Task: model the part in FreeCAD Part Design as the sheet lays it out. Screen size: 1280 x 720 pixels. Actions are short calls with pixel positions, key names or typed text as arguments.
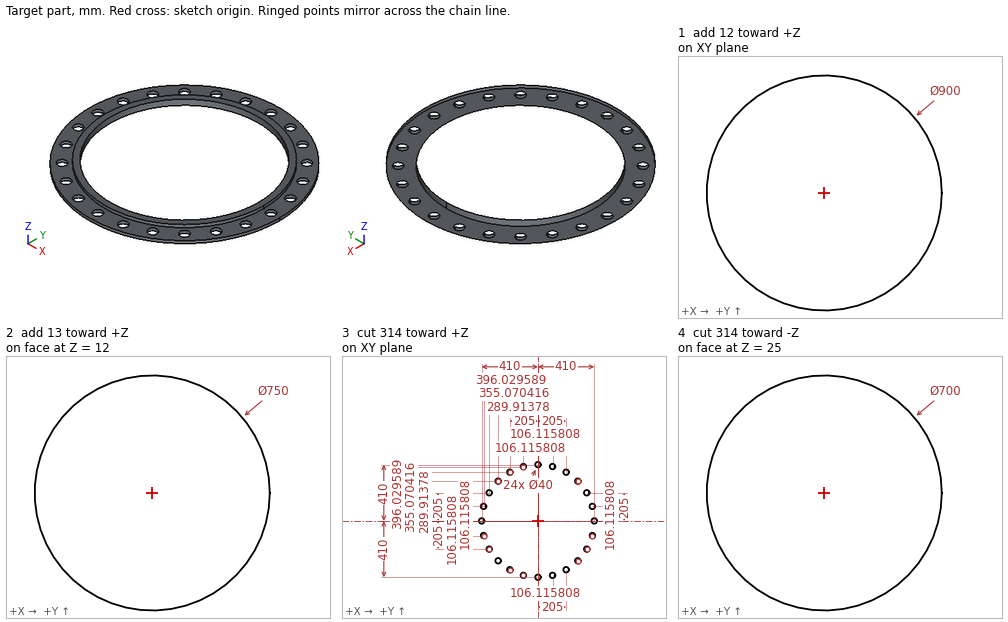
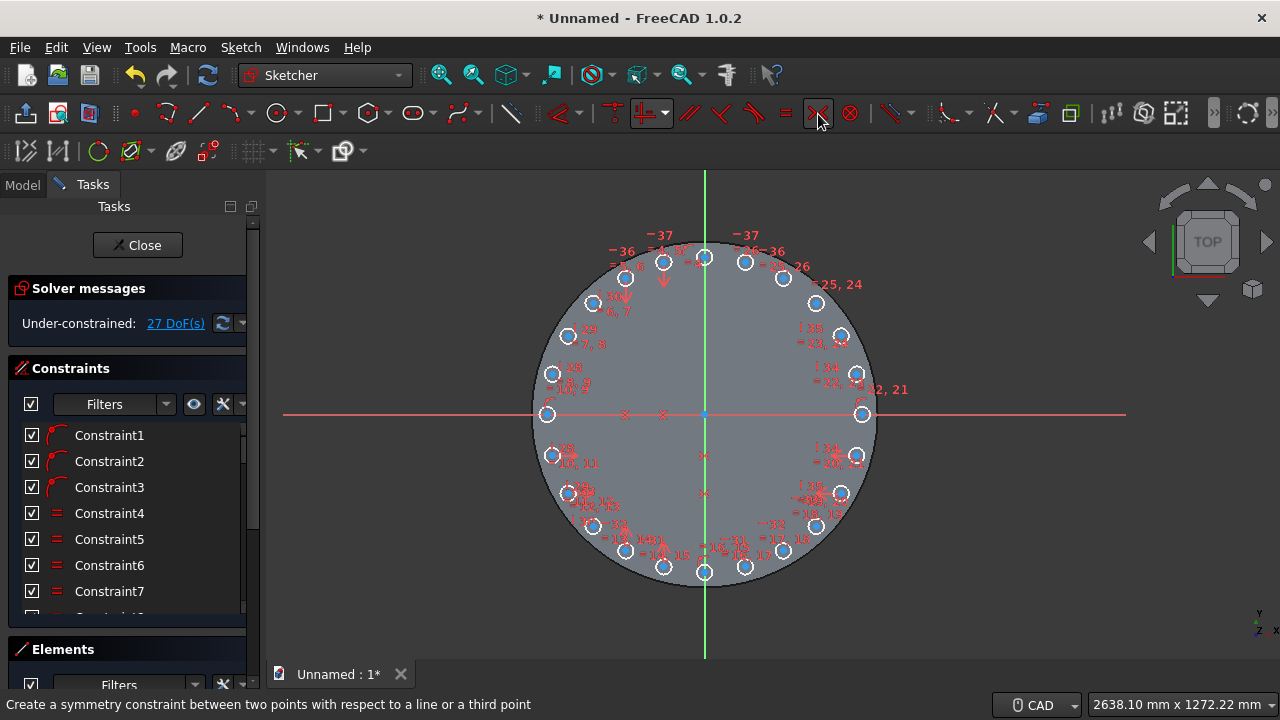
click(593, 303)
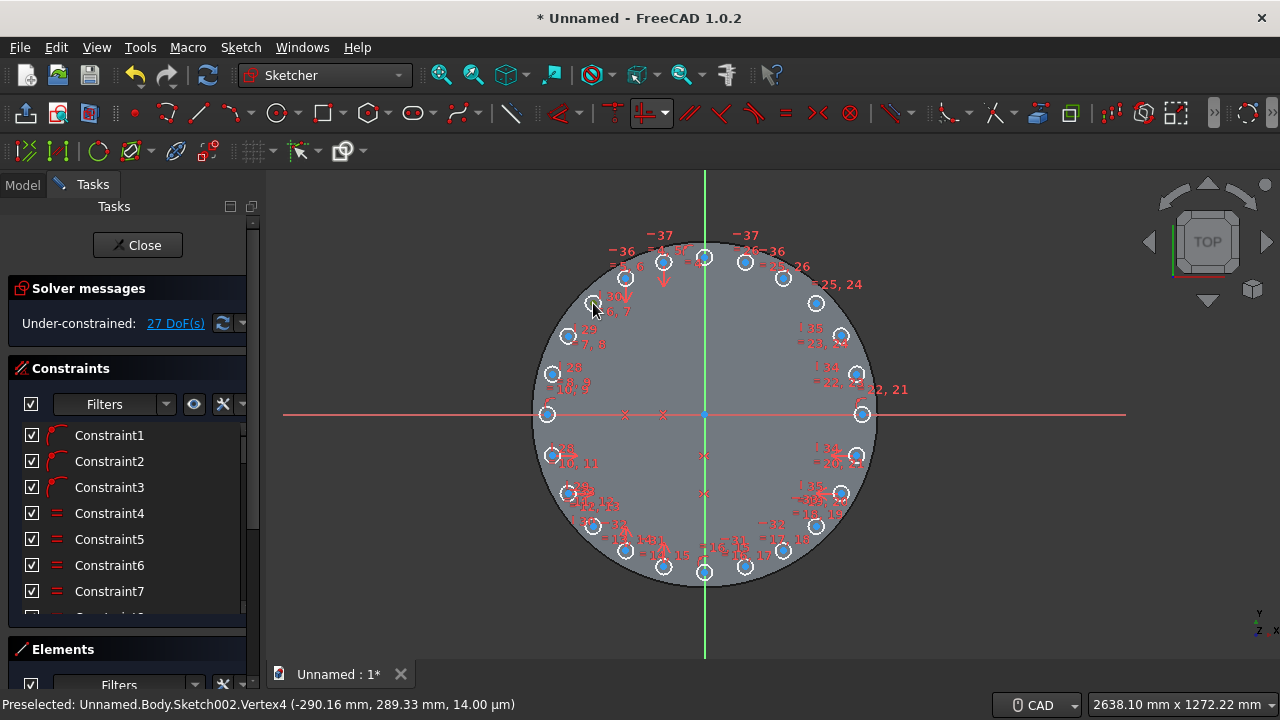
click(816, 303)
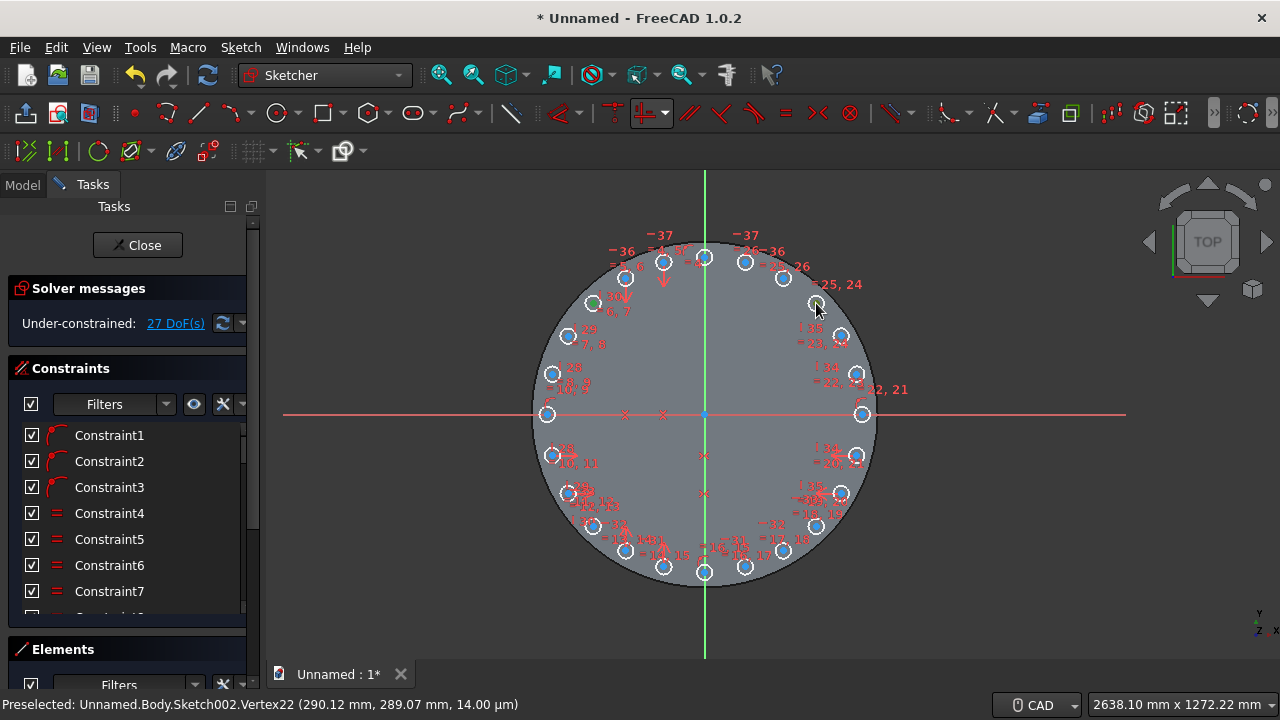
click(705, 507)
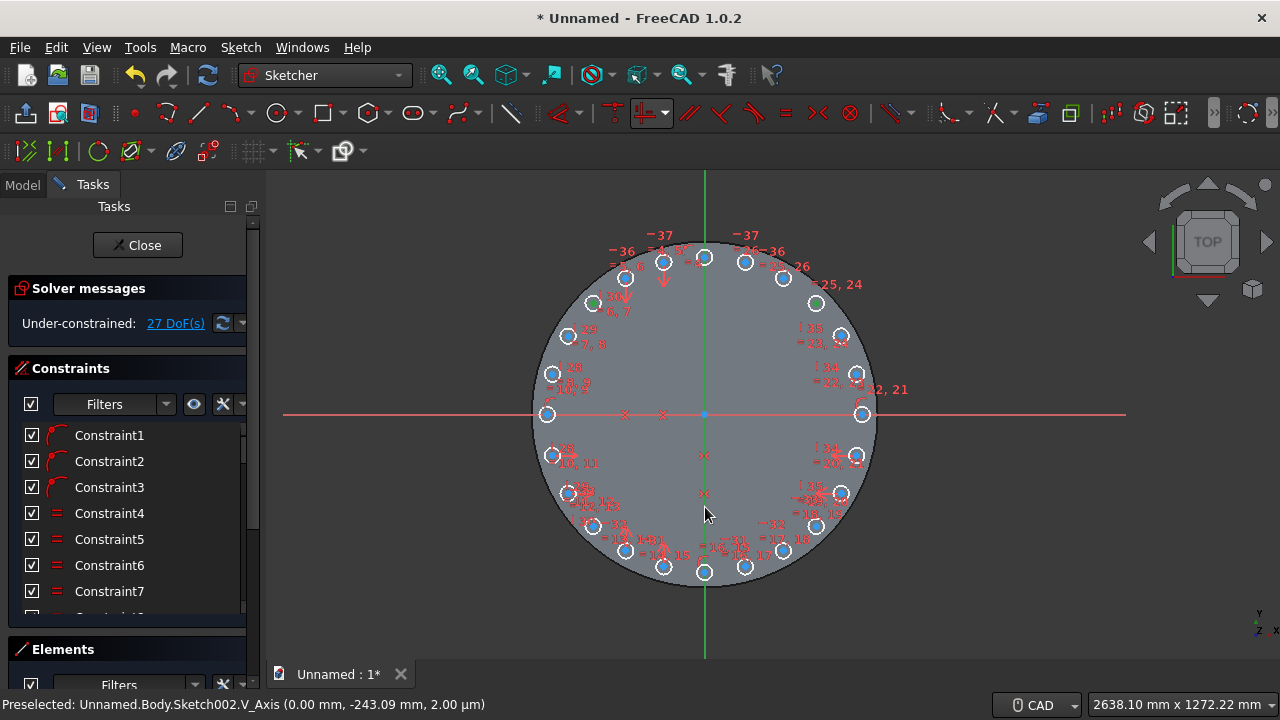
click(818, 114)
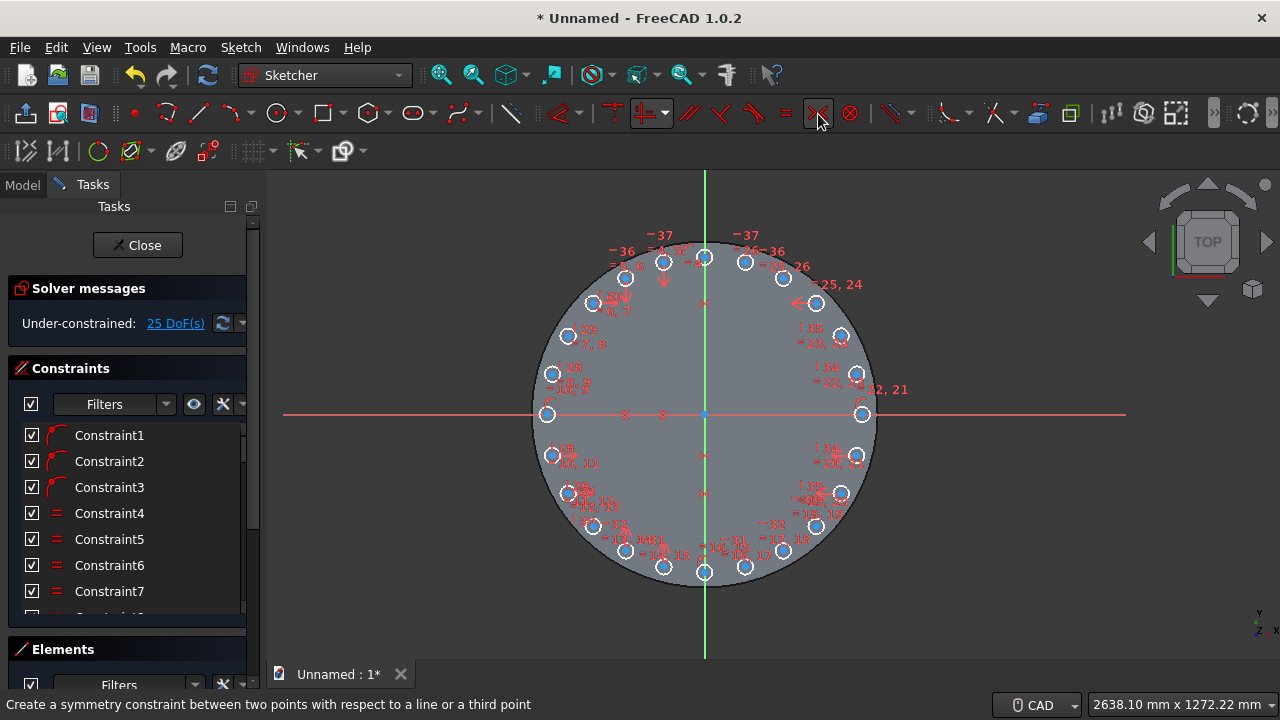
click(816, 526)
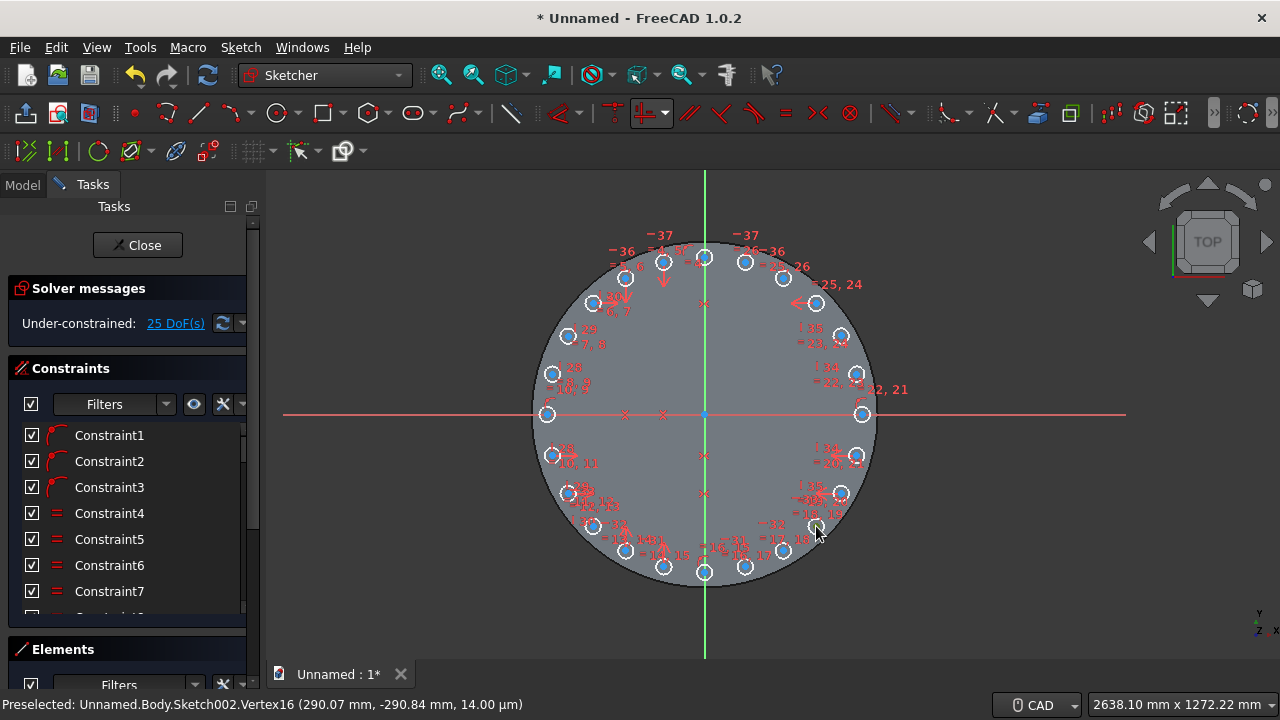
click(816, 303)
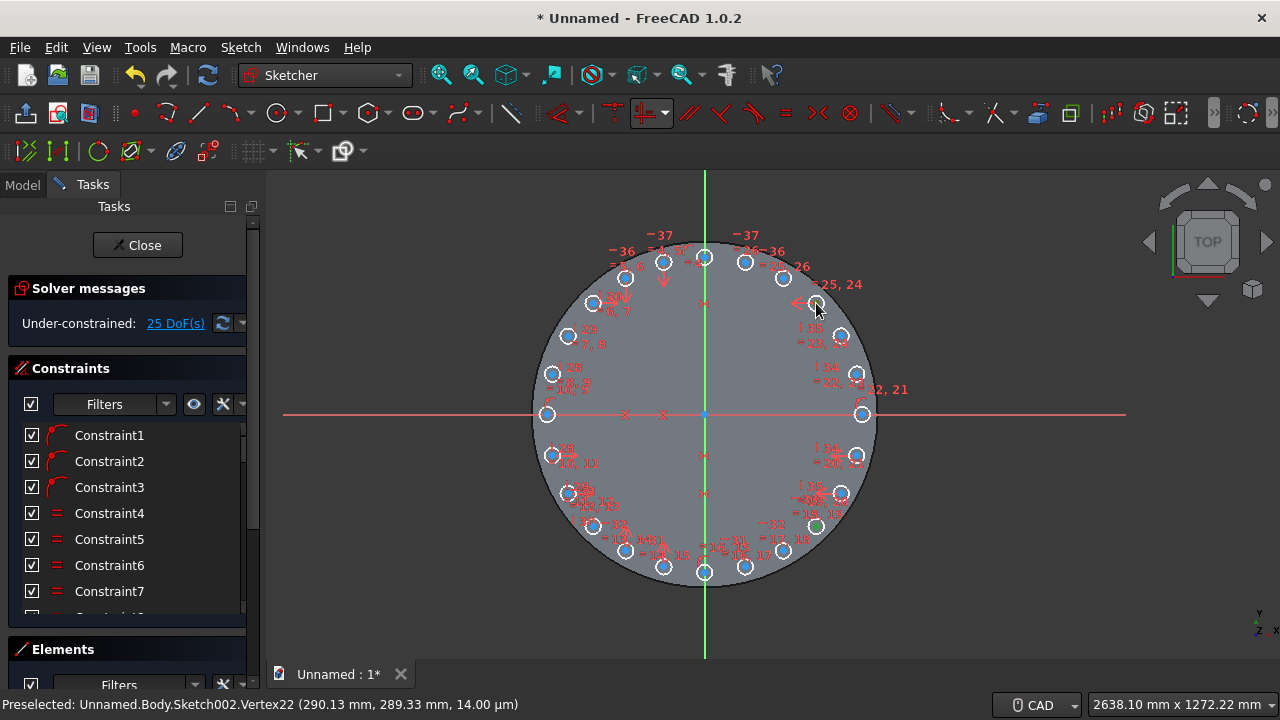
click(353, 415)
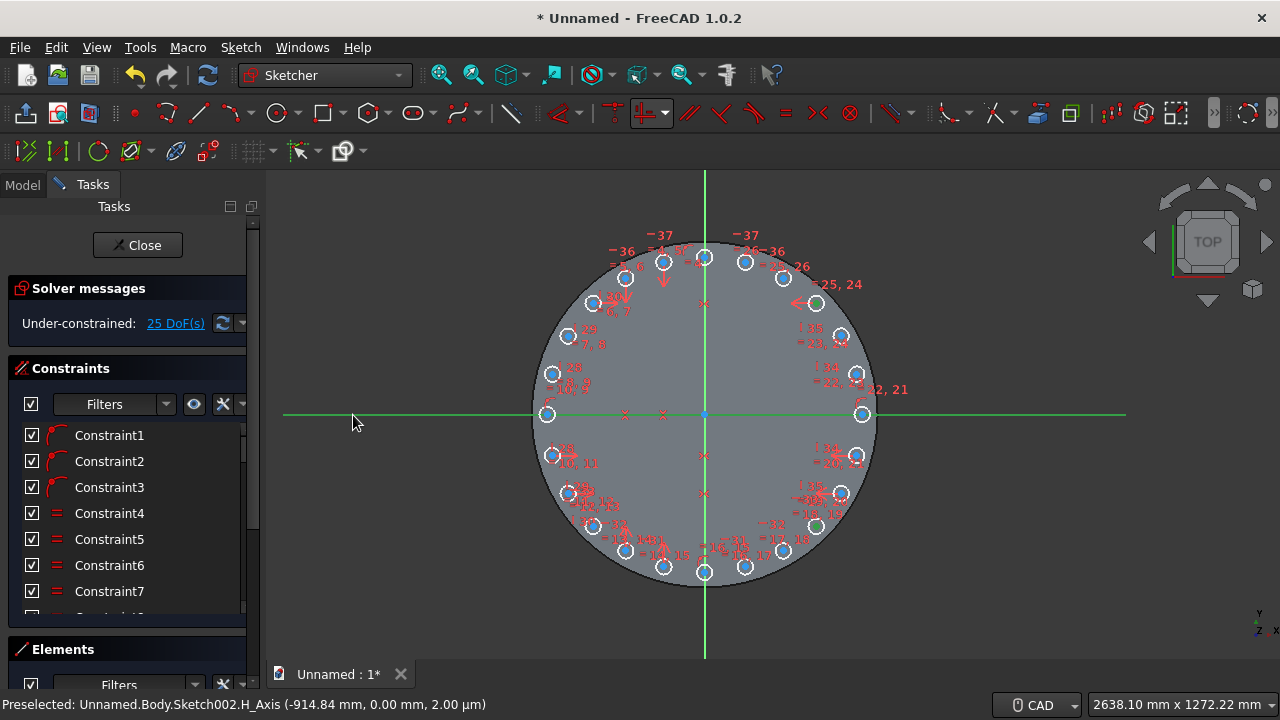
click(818, 114)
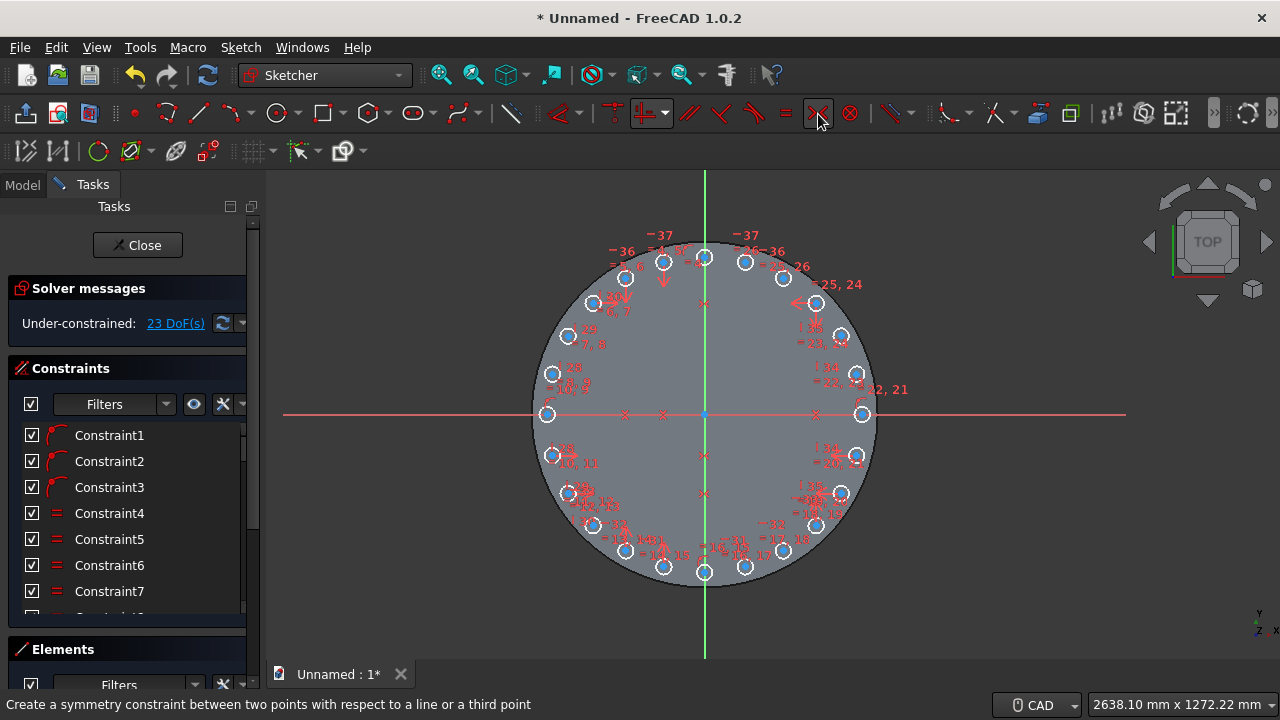
click(558, 114)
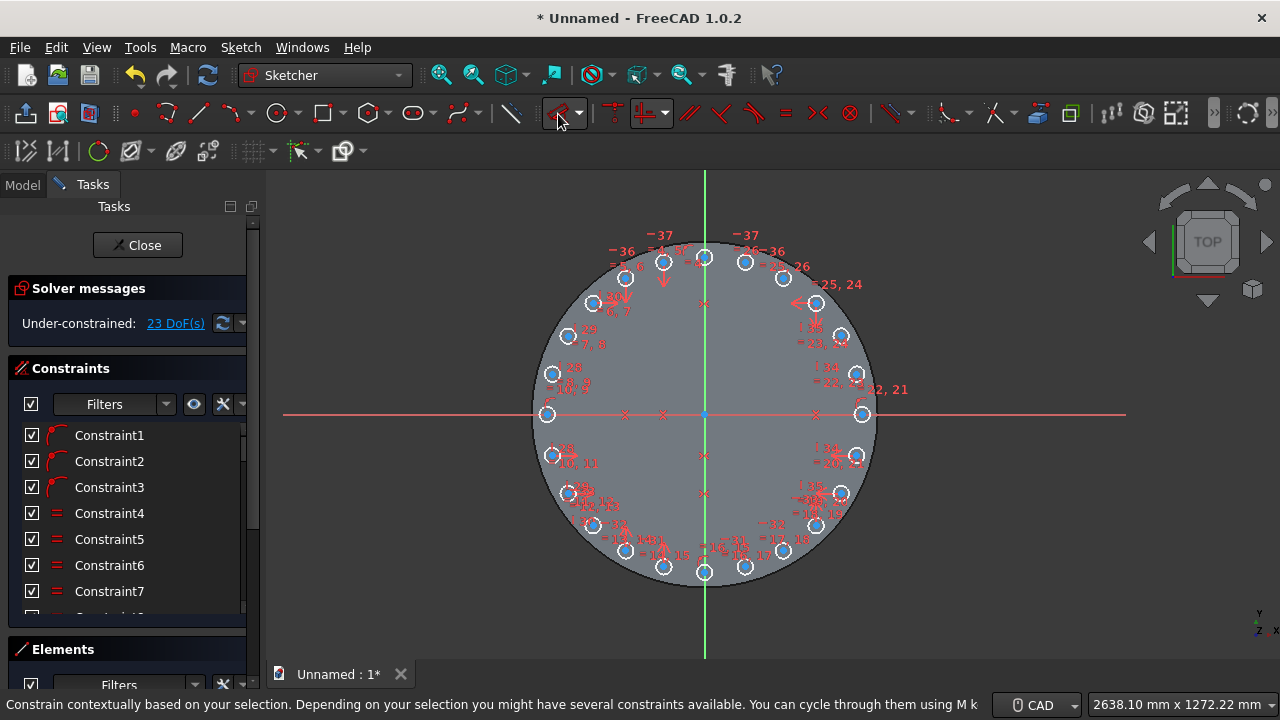
scroll(705, 250, up, 5)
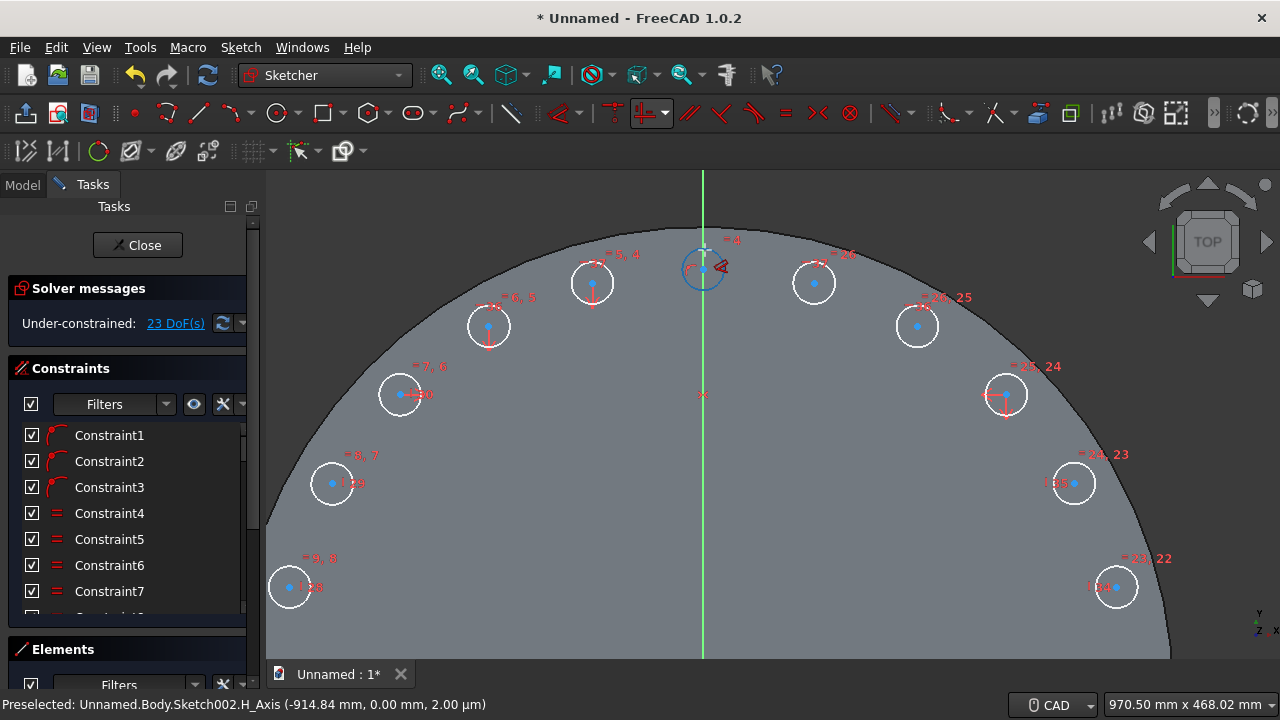
click(704, 249)
click(730, 224)